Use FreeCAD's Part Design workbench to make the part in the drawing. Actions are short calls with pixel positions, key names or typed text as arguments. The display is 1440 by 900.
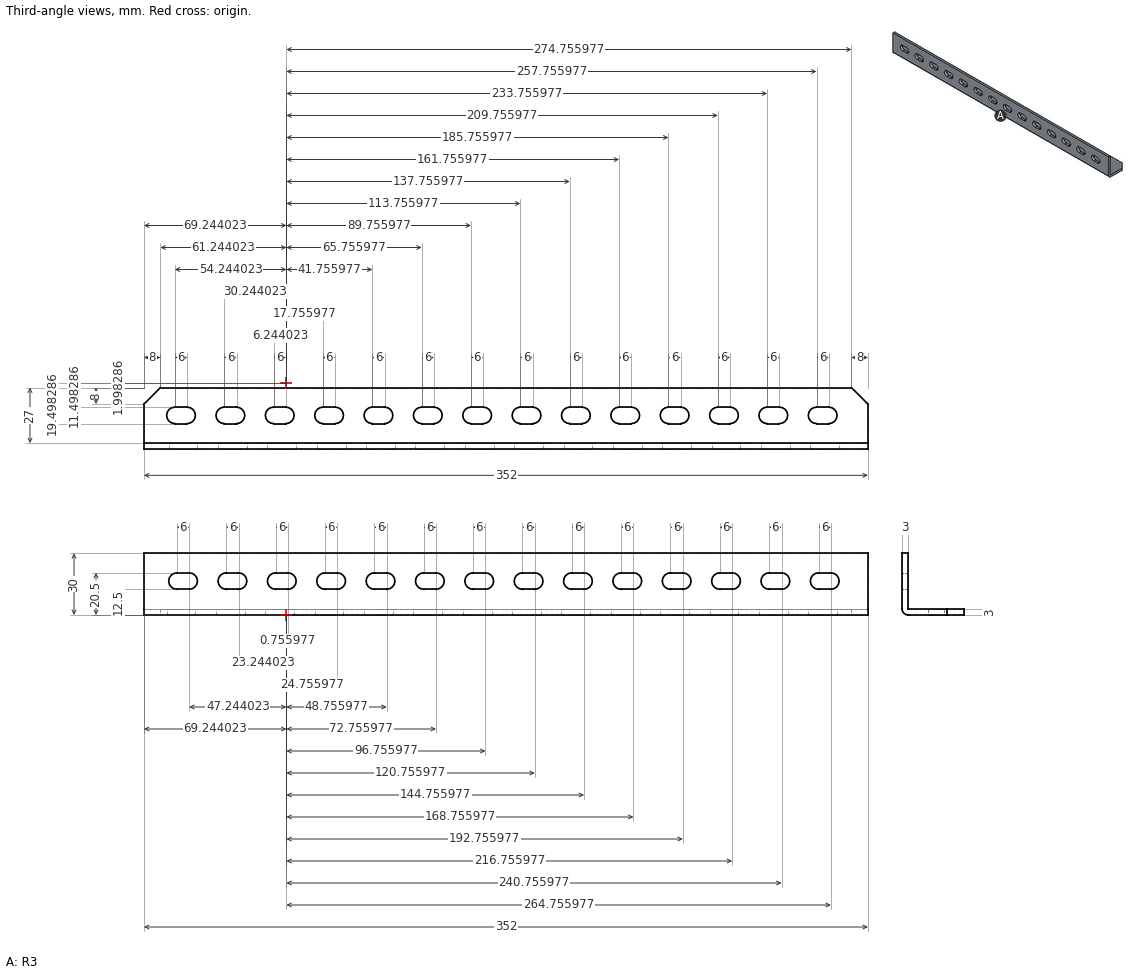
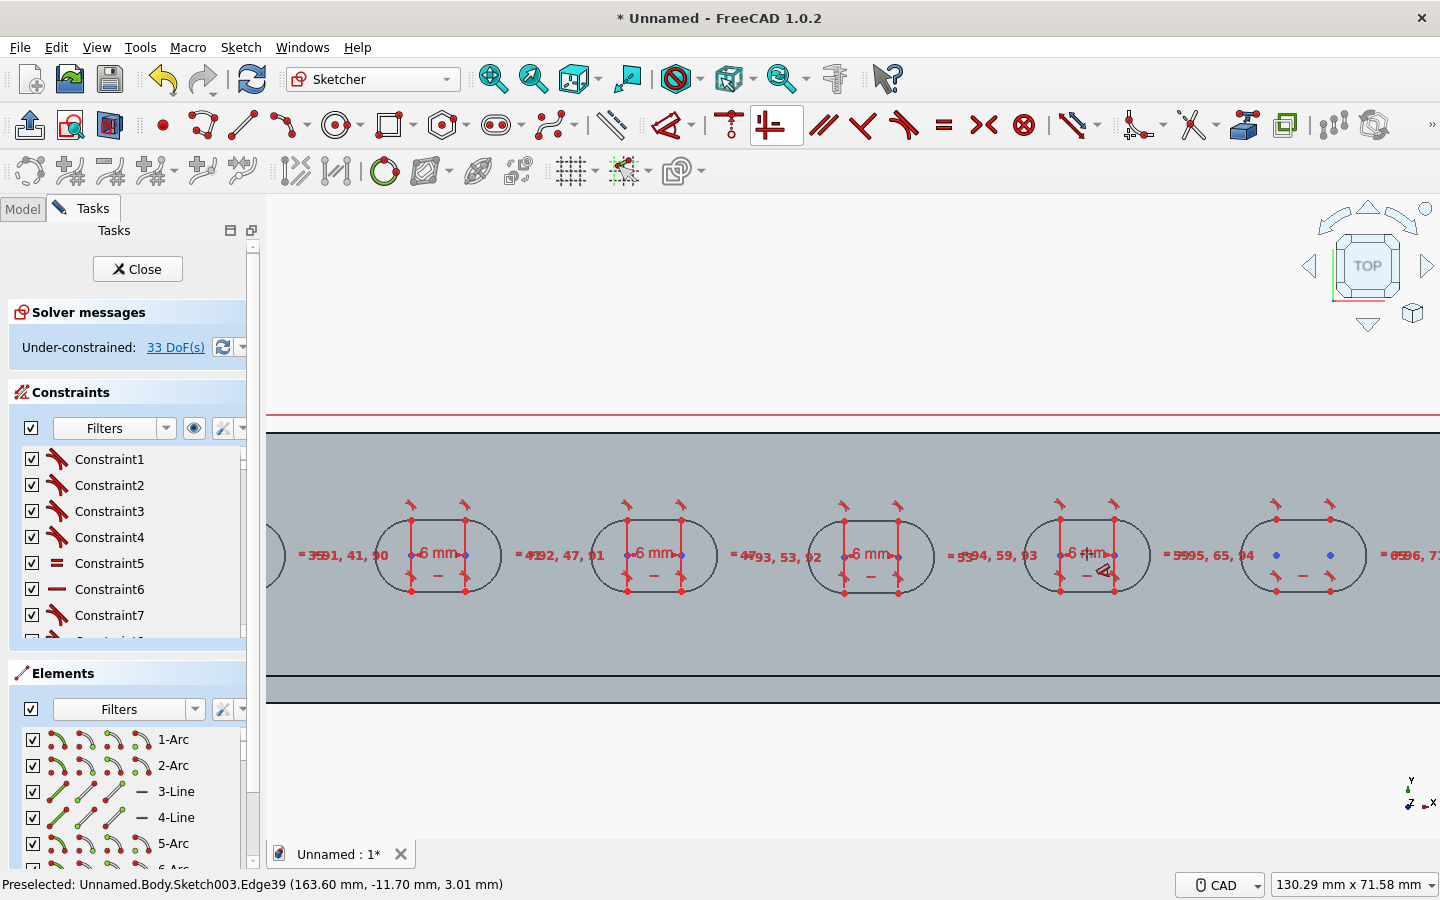
scroll(862, 521, down, 7)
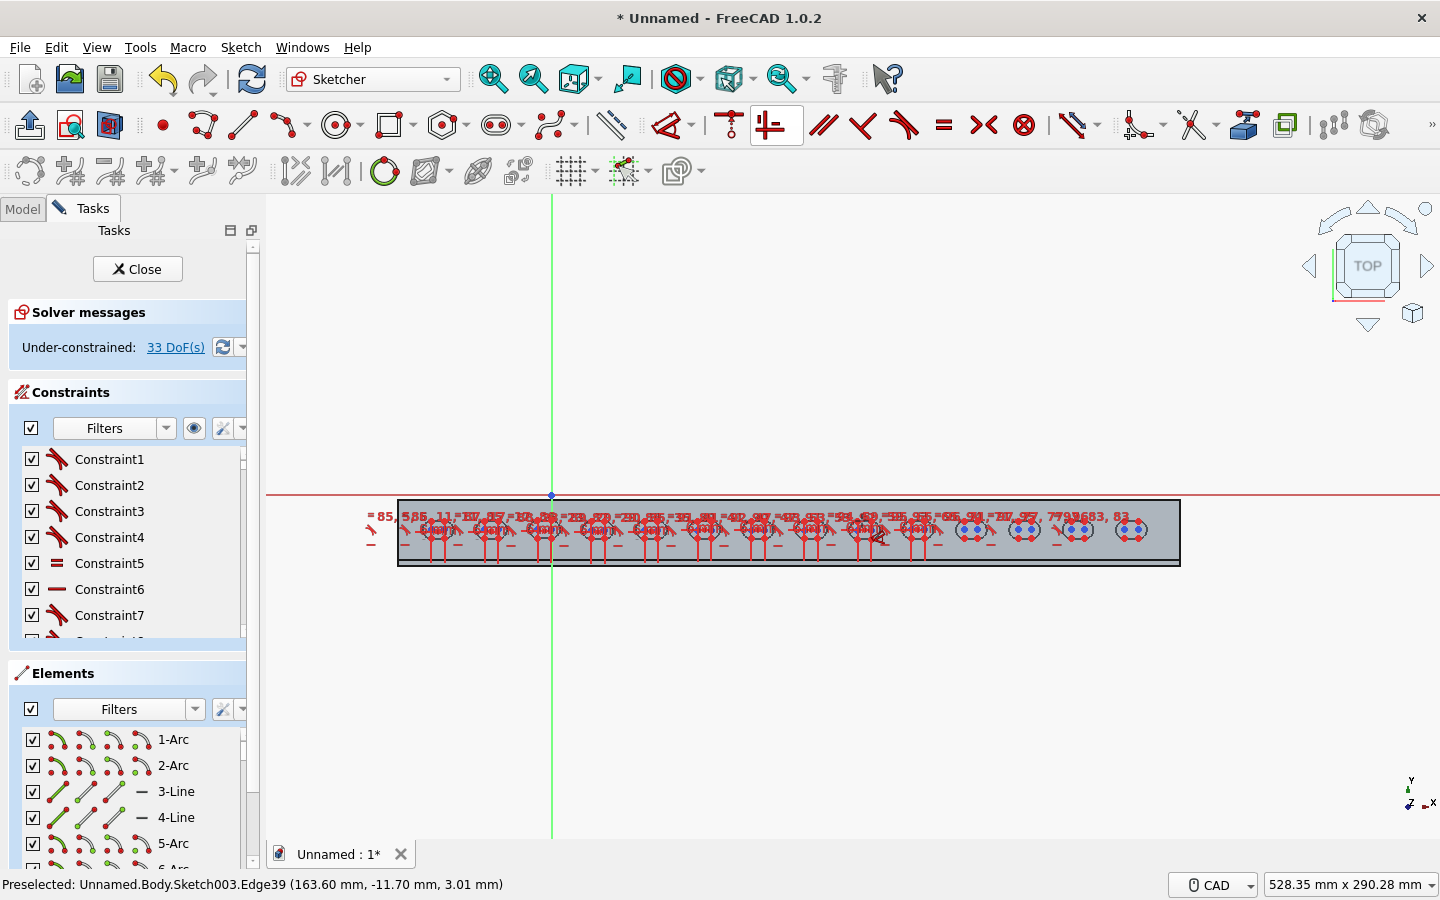
scroll(969, 521, up, 7)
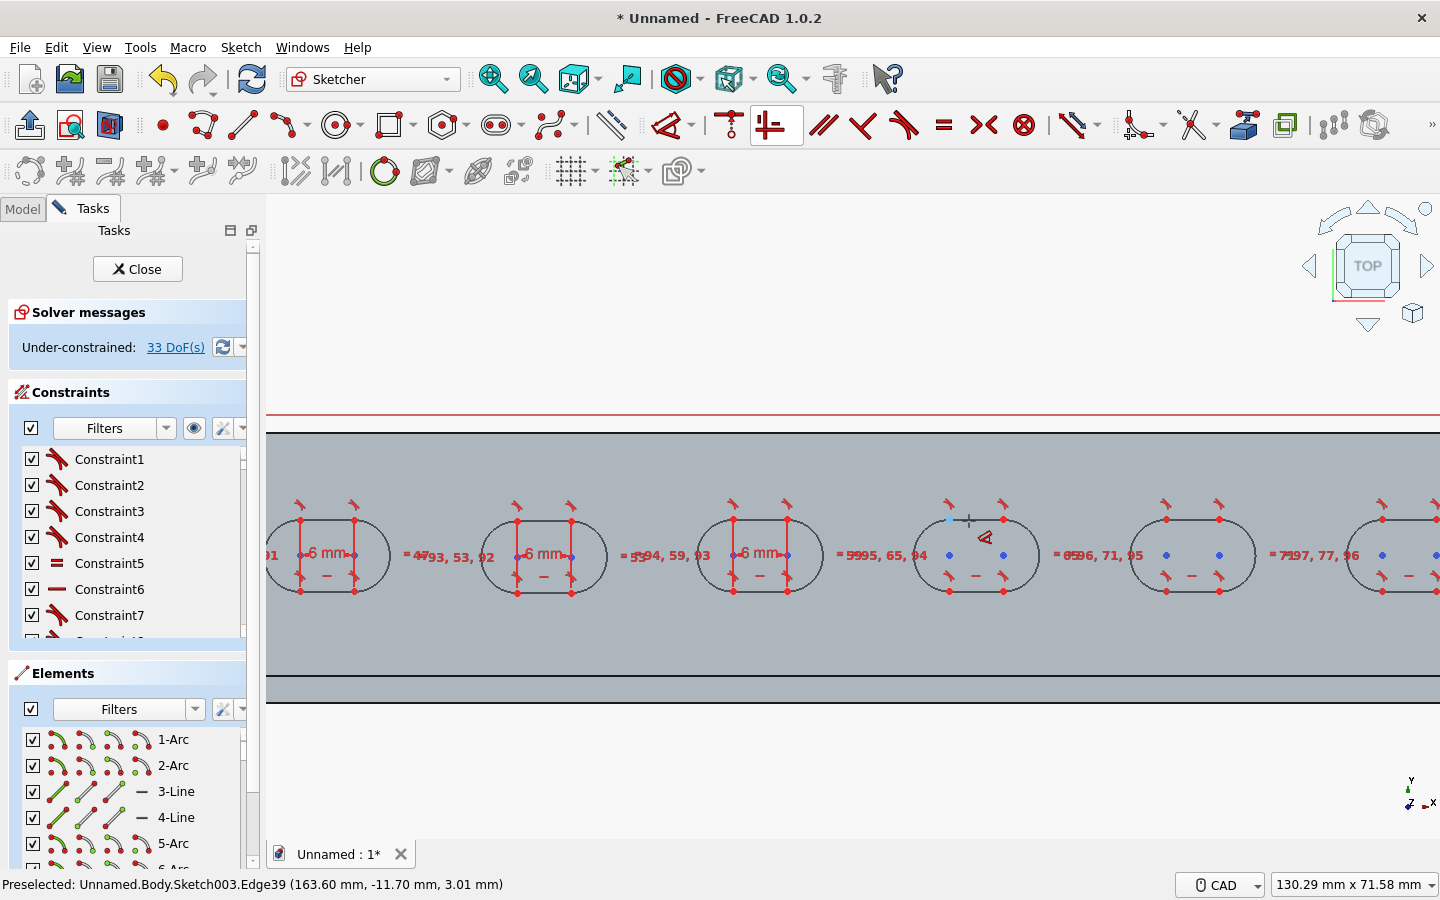
click(966, 520)
click(977, 554)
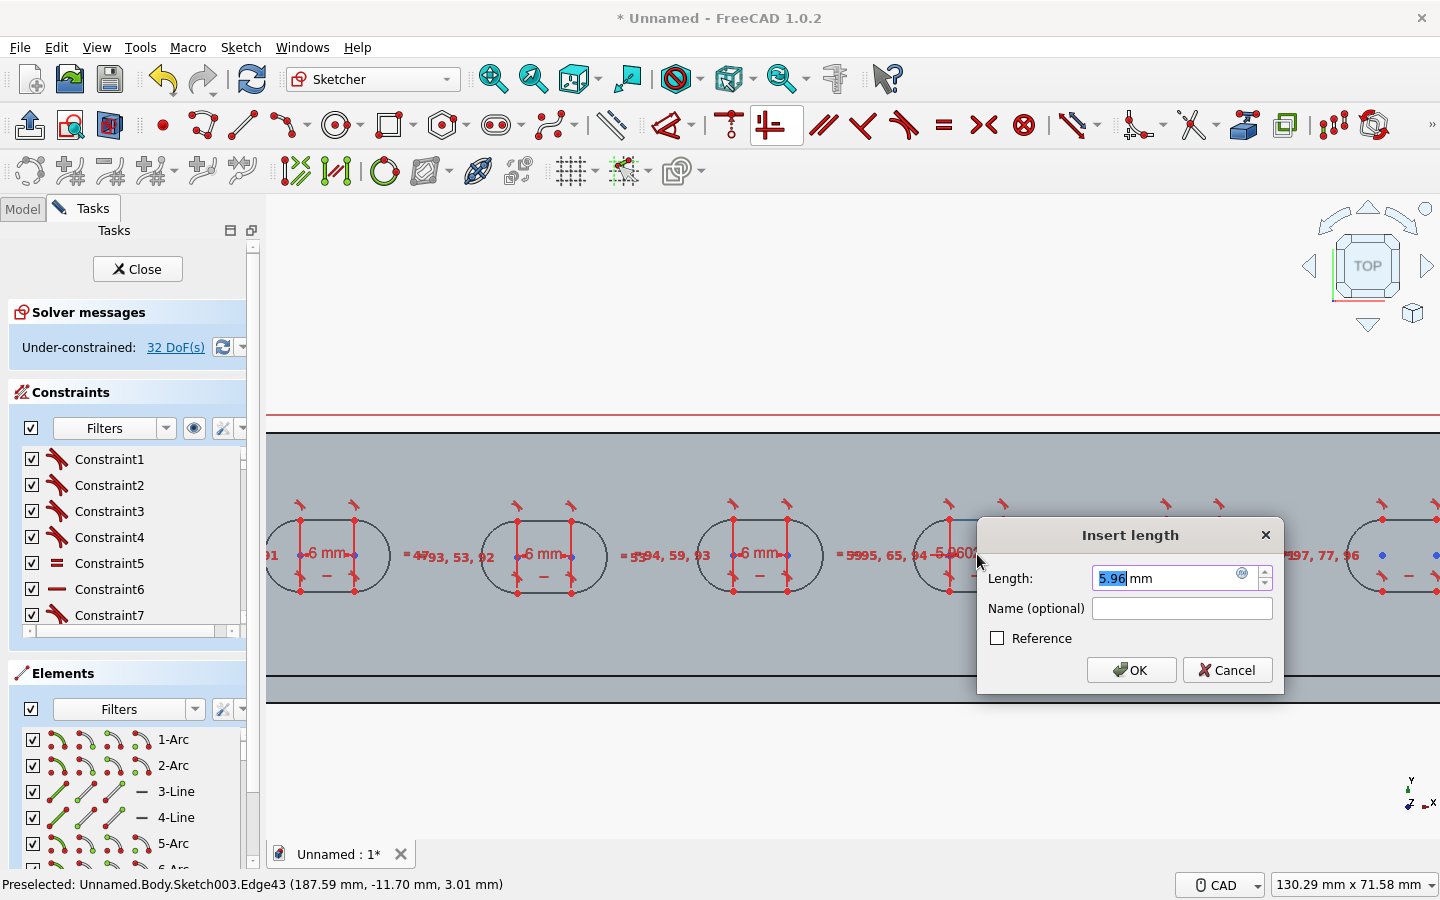
text(6)
key(Return)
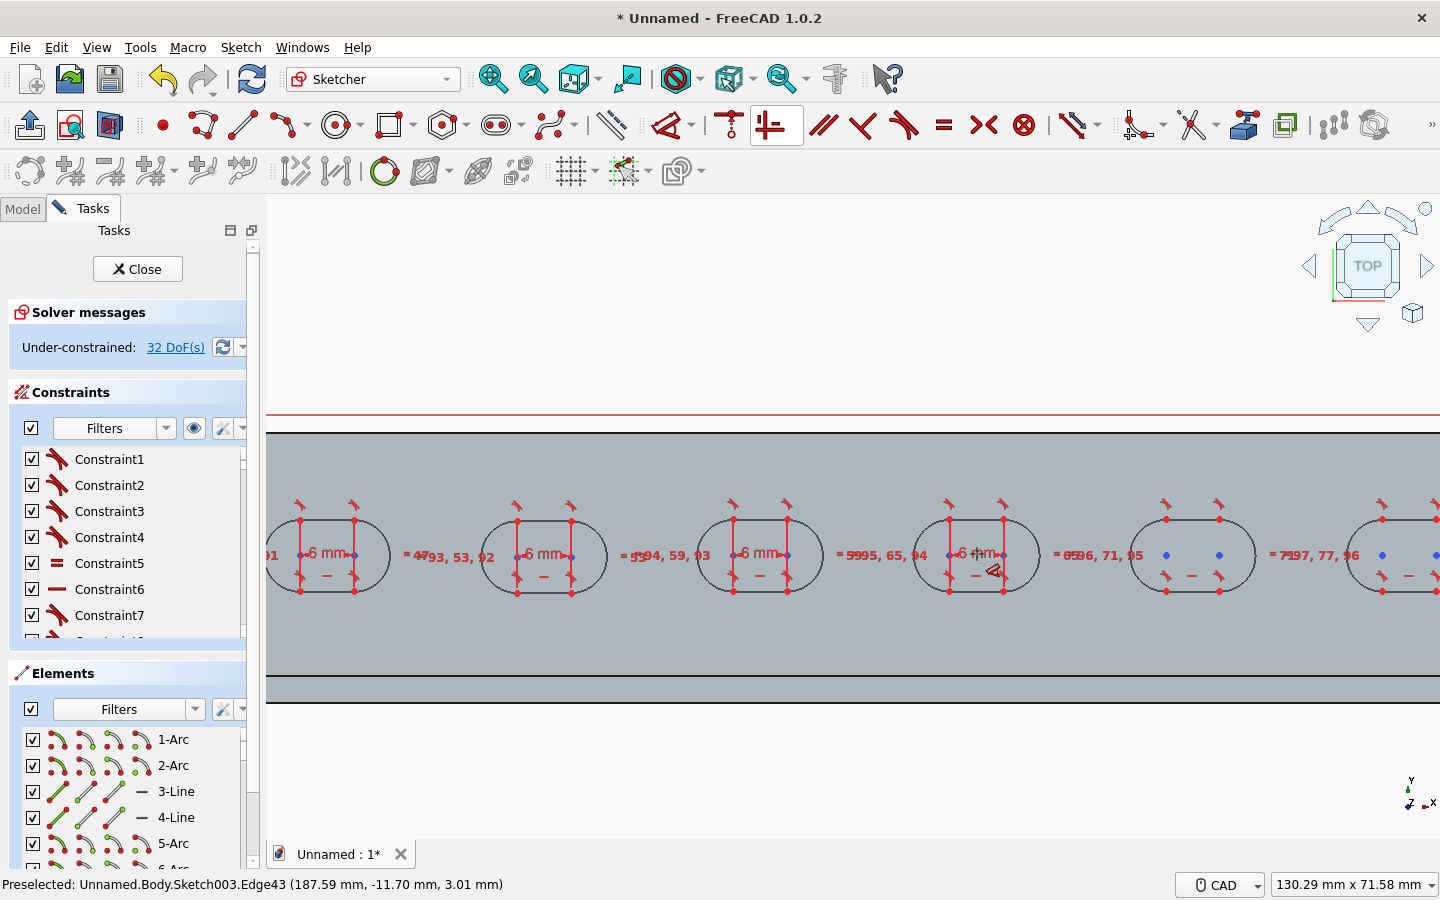
click(1182, 520)
click(1193, 554)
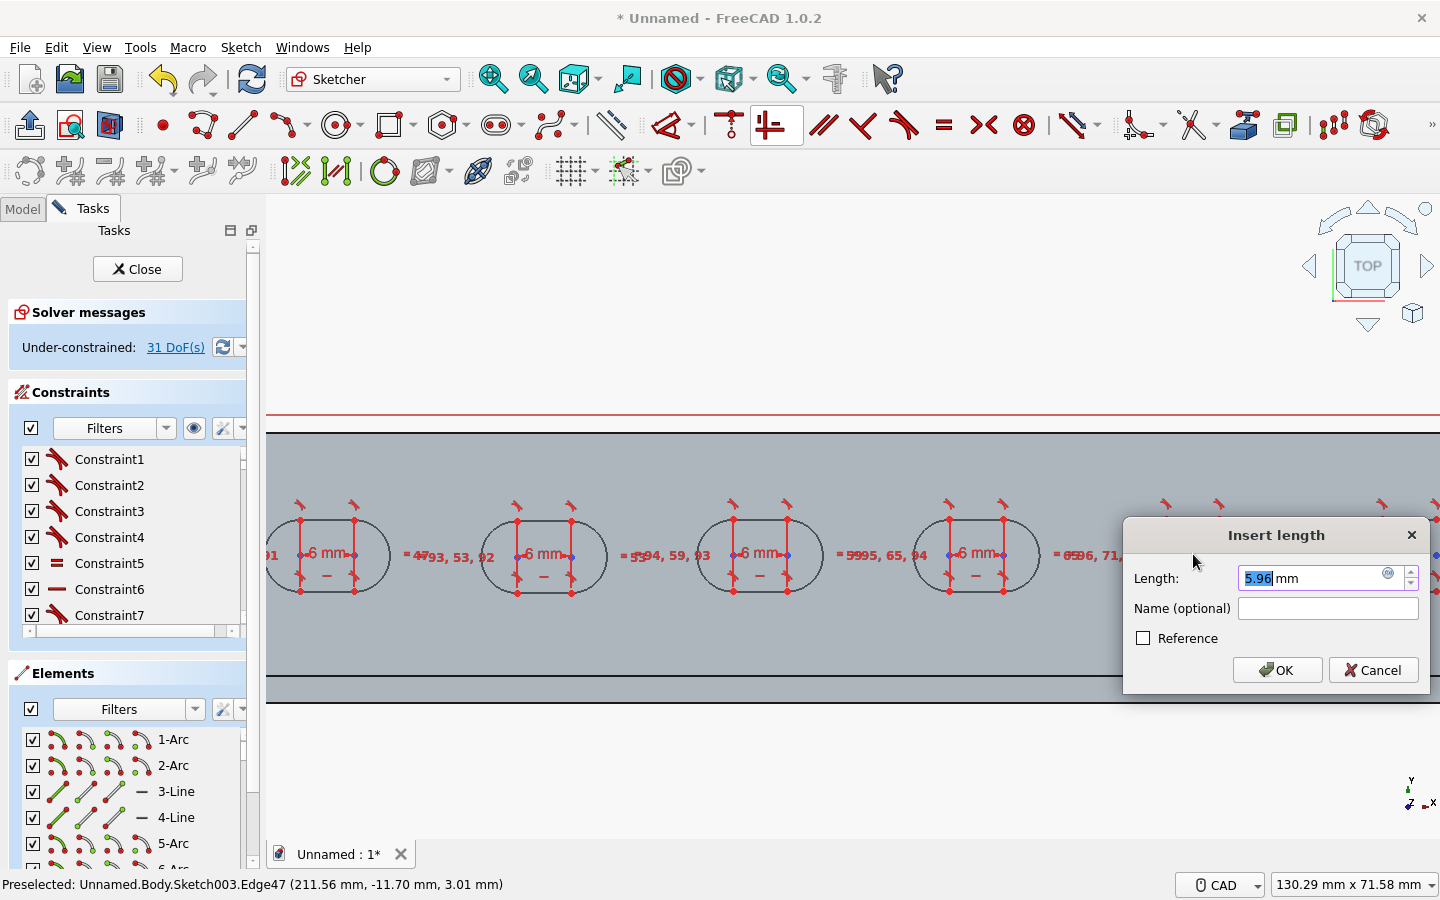
text(6)
key(Return)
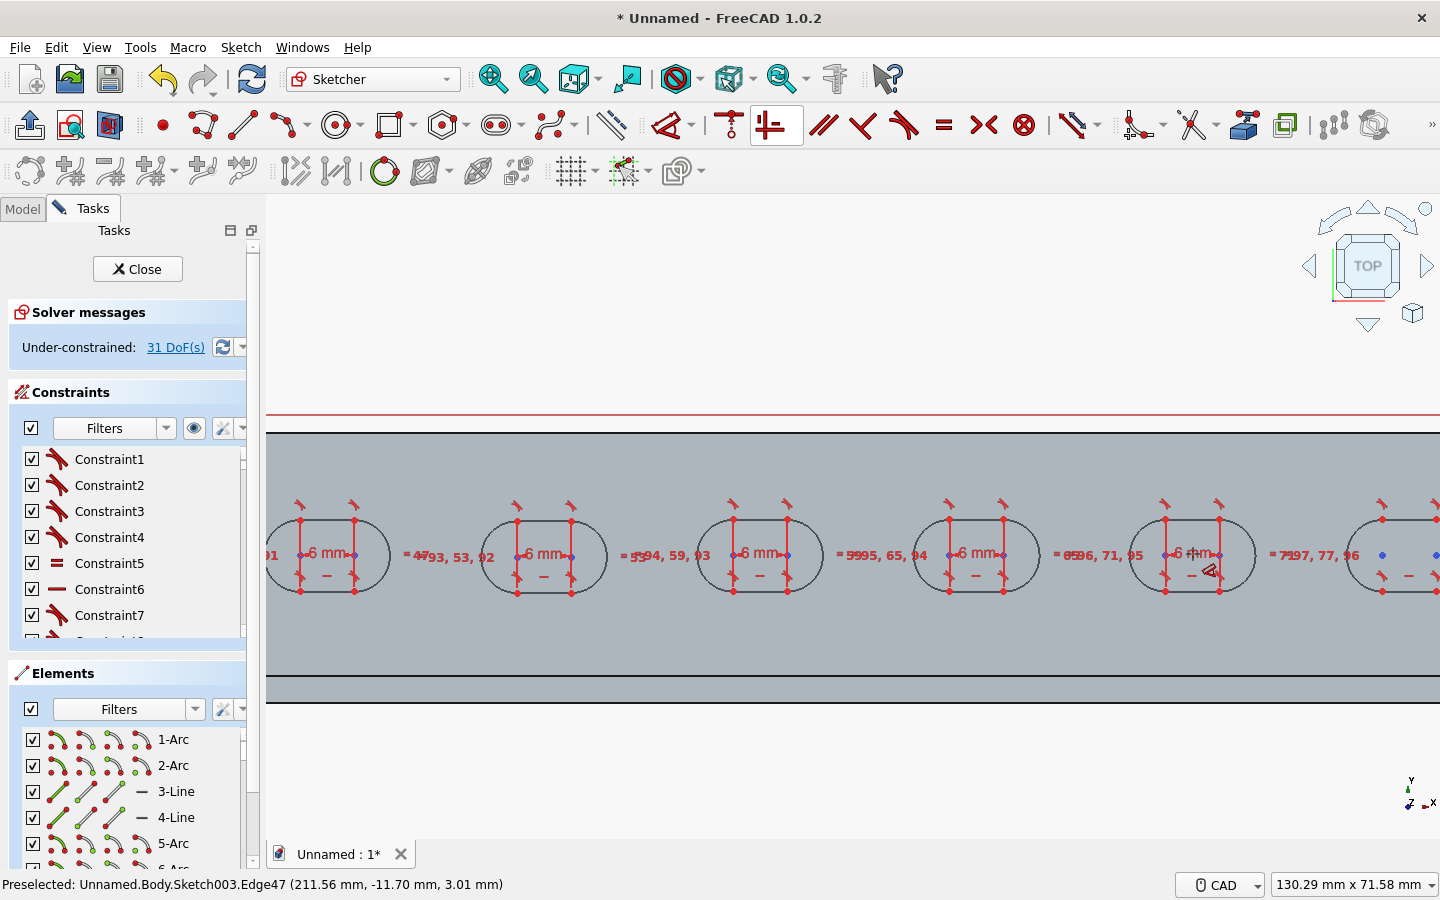
scroll(969, 521, down, 7)